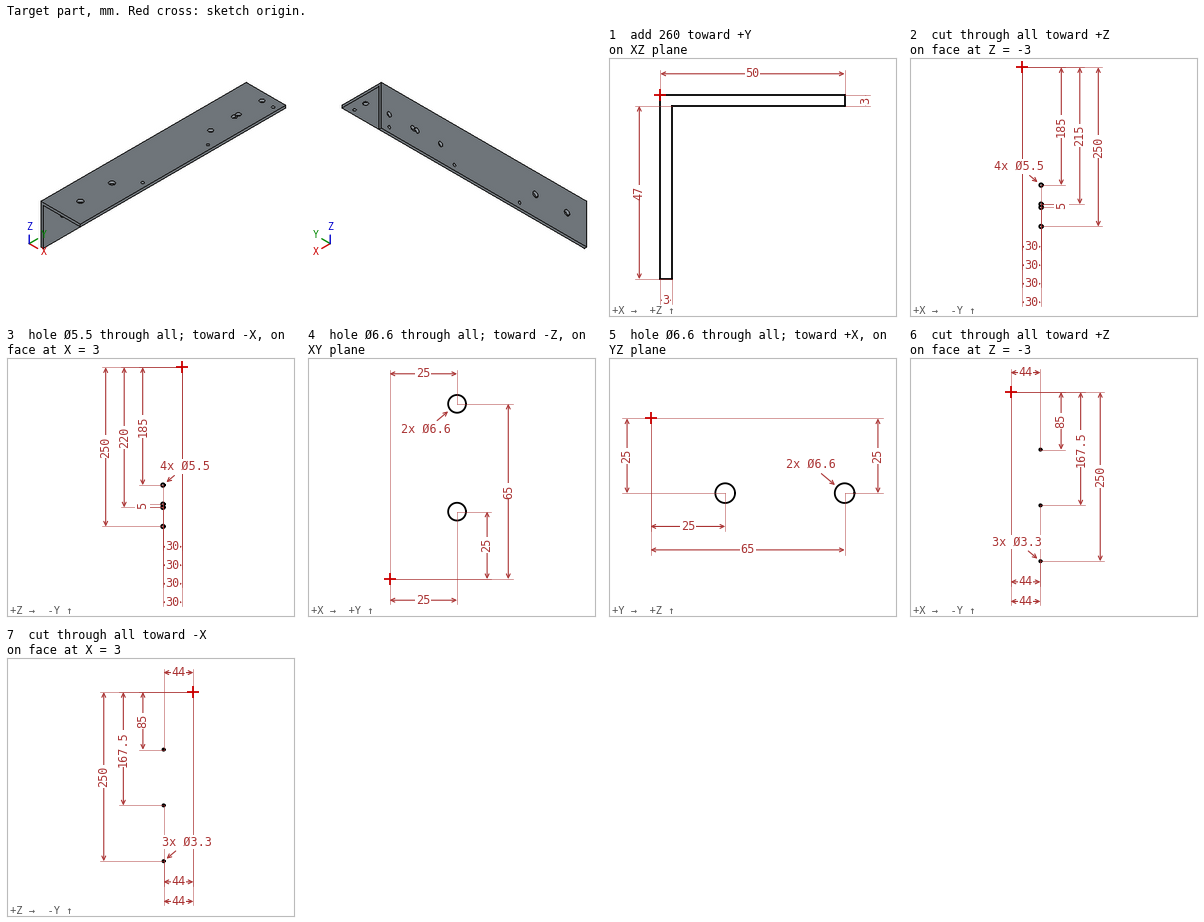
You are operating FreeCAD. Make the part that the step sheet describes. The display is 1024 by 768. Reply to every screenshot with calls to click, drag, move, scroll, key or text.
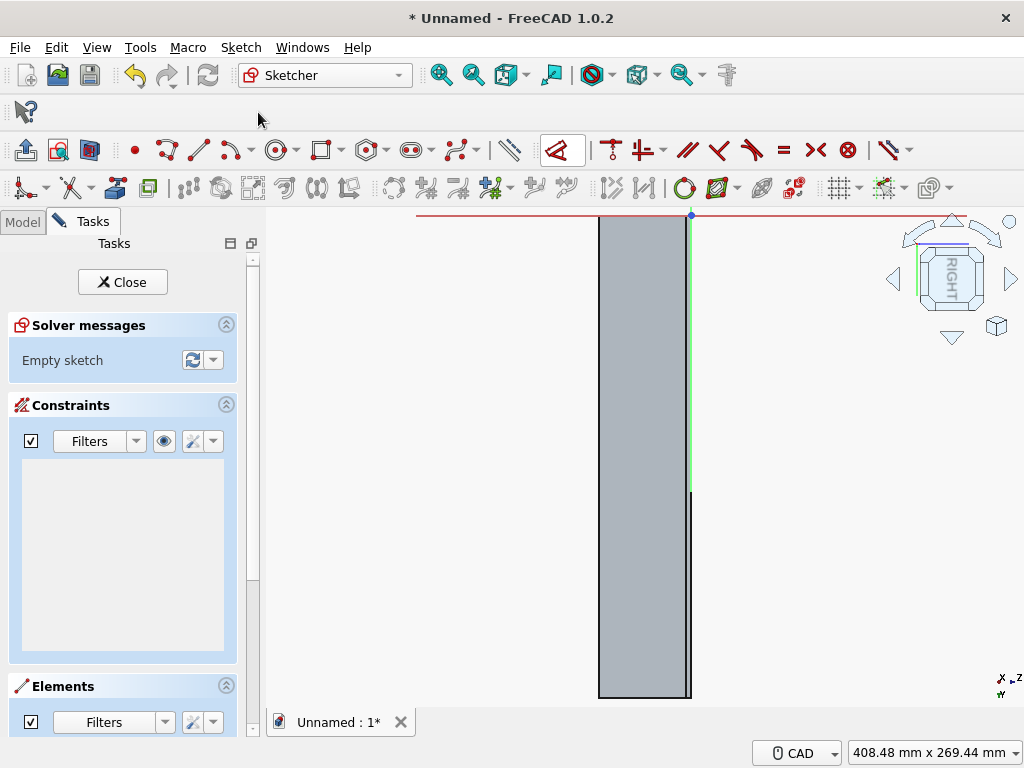
scroll(576, 457, down, 5)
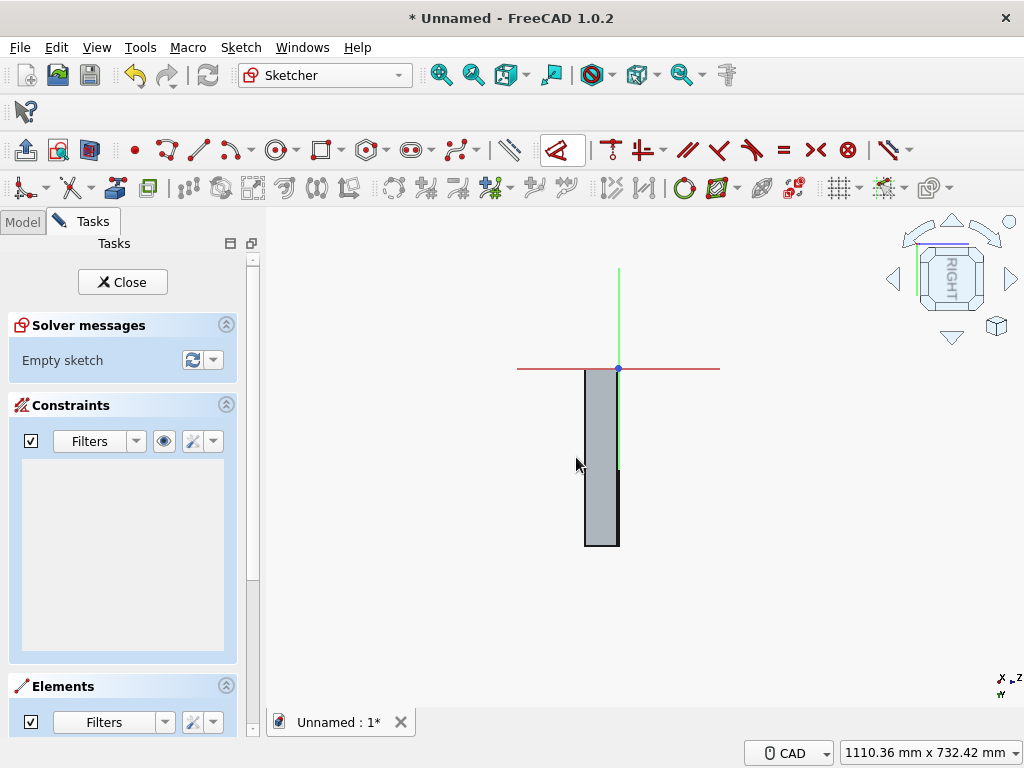
scroll(603, 529, up, 9)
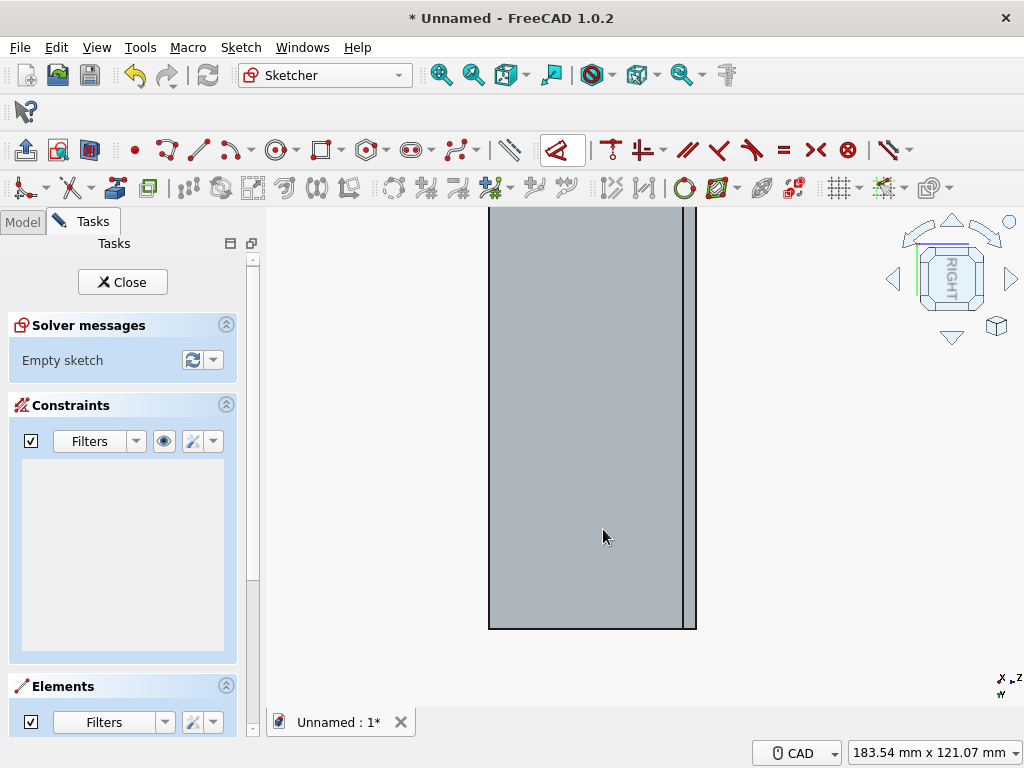
key(g)
key(c)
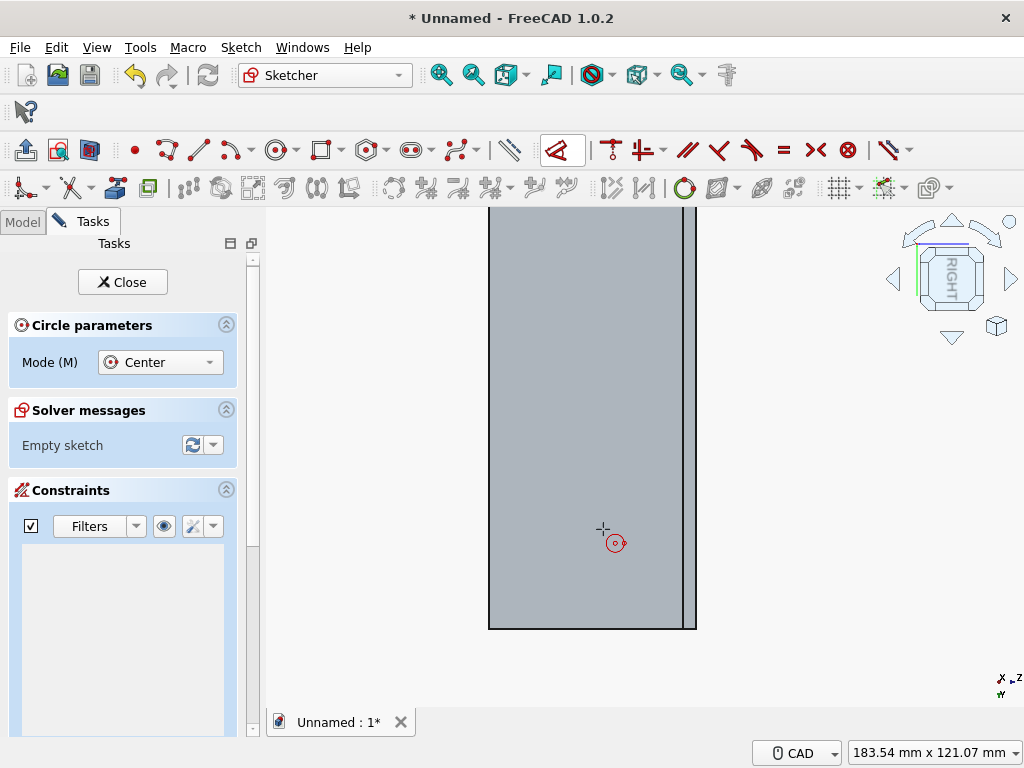
scroll(572, 464, up, 4)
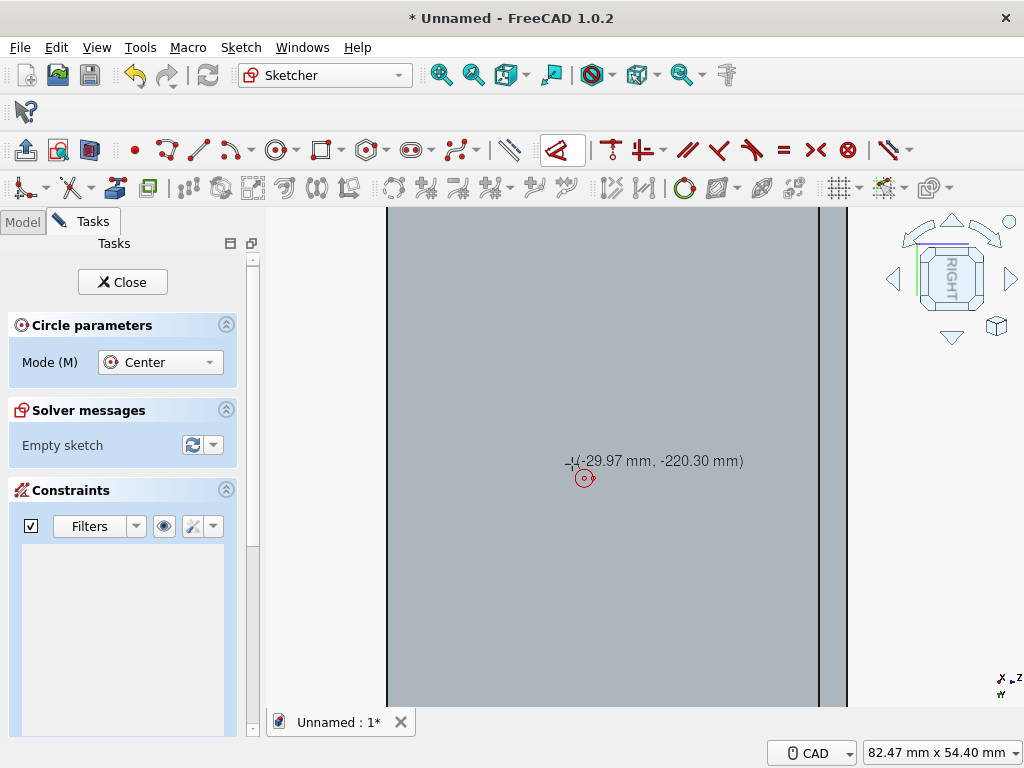
click(571, 463)
click(589, 445)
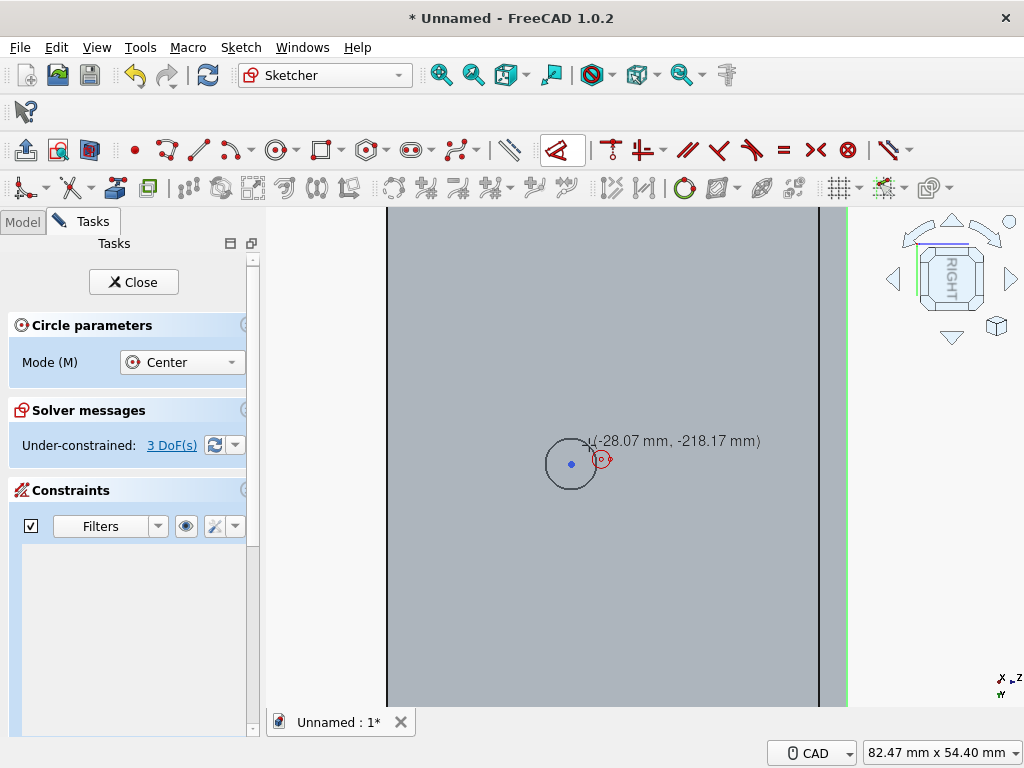
scroll(581, 471, down, 4)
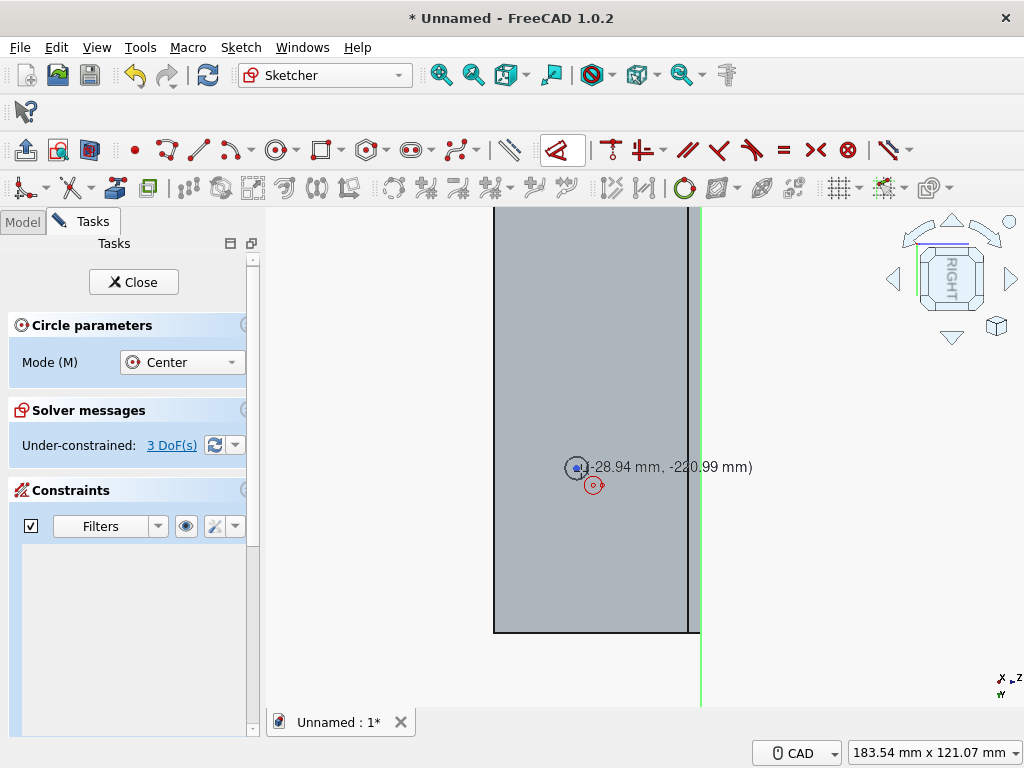
scroll(577, 323, up, 4)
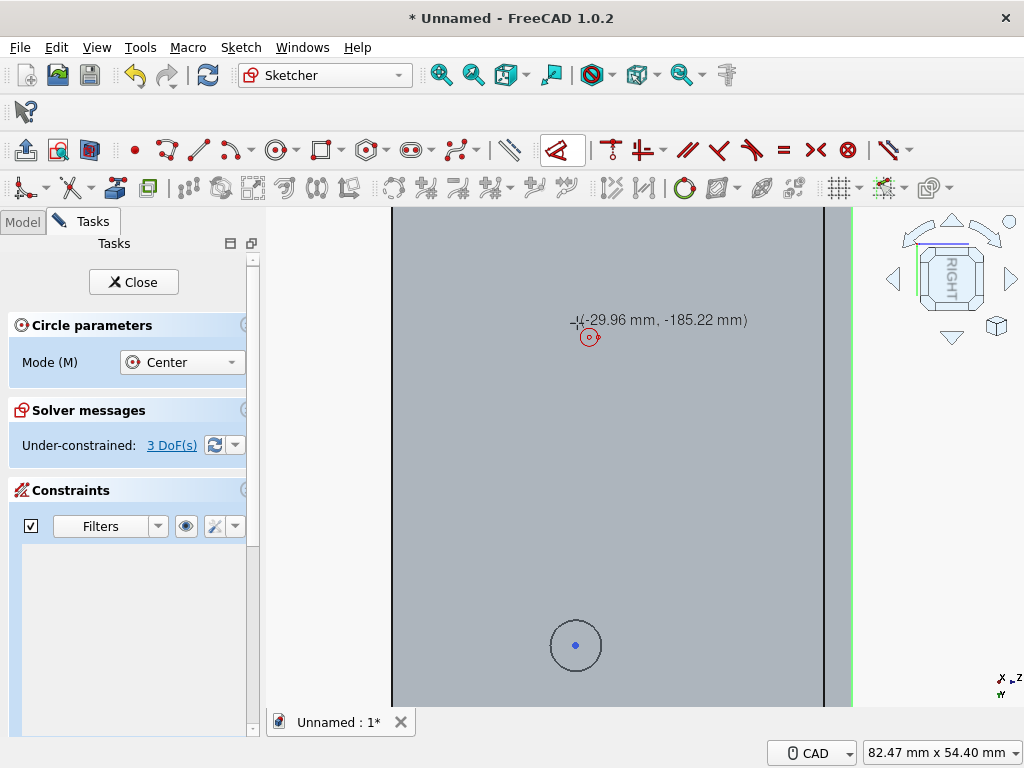
click(576, 323)
click(594, 305)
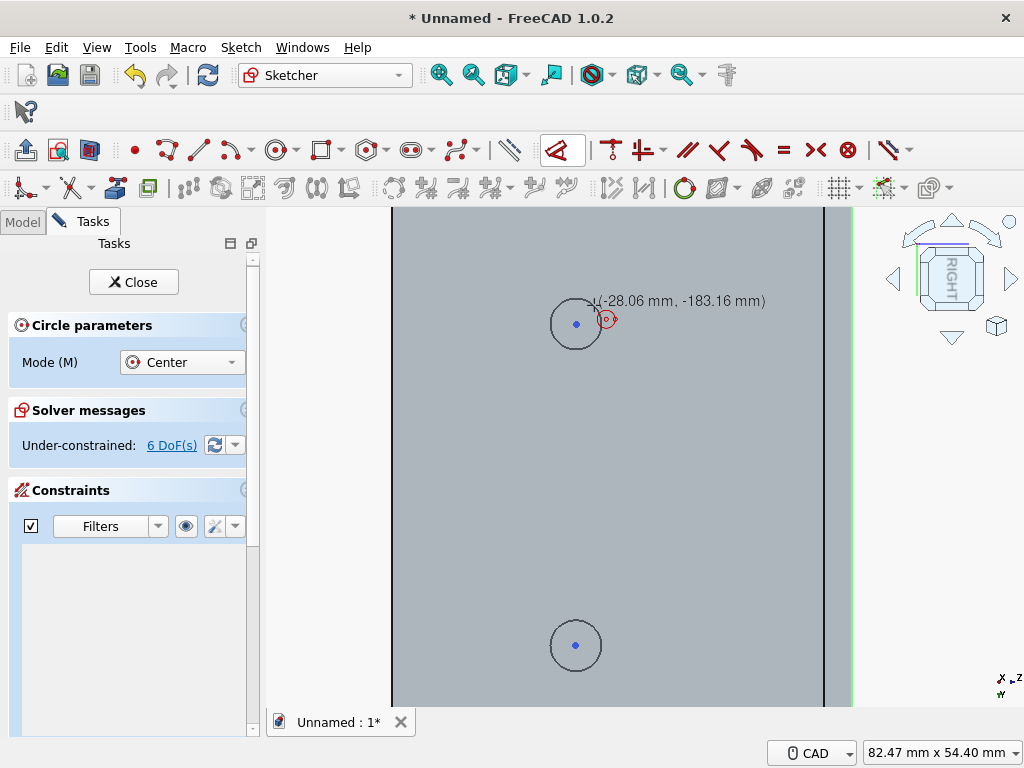
scroll(577, 323, down, 4)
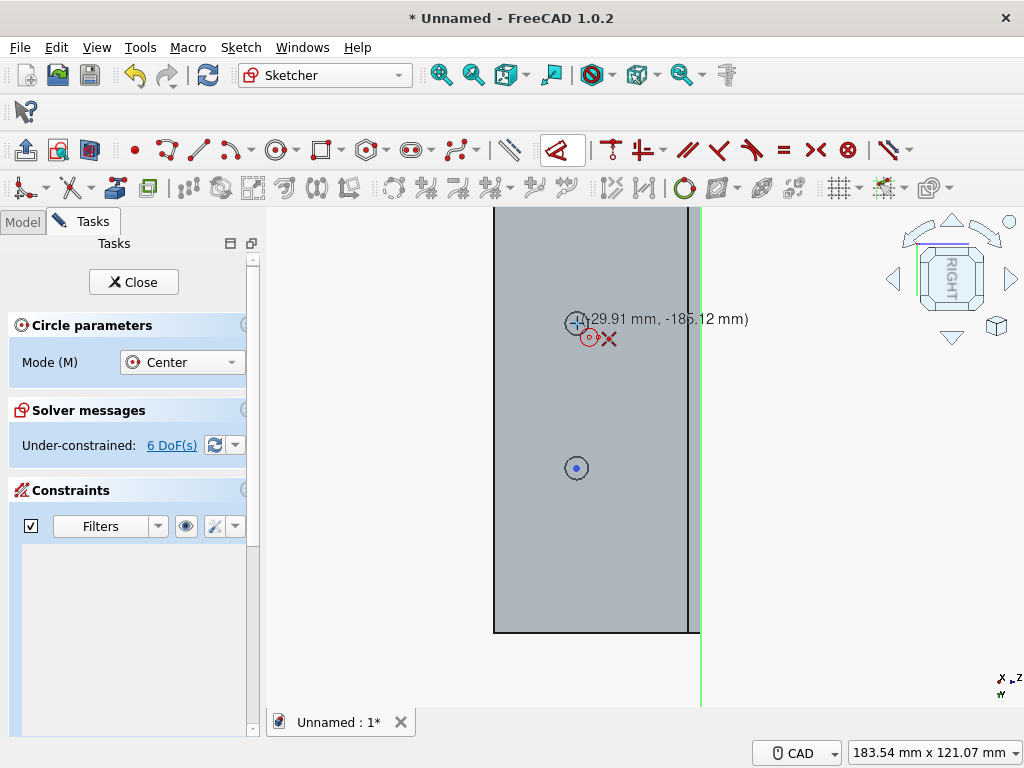
scroll(577, 592, up, 4)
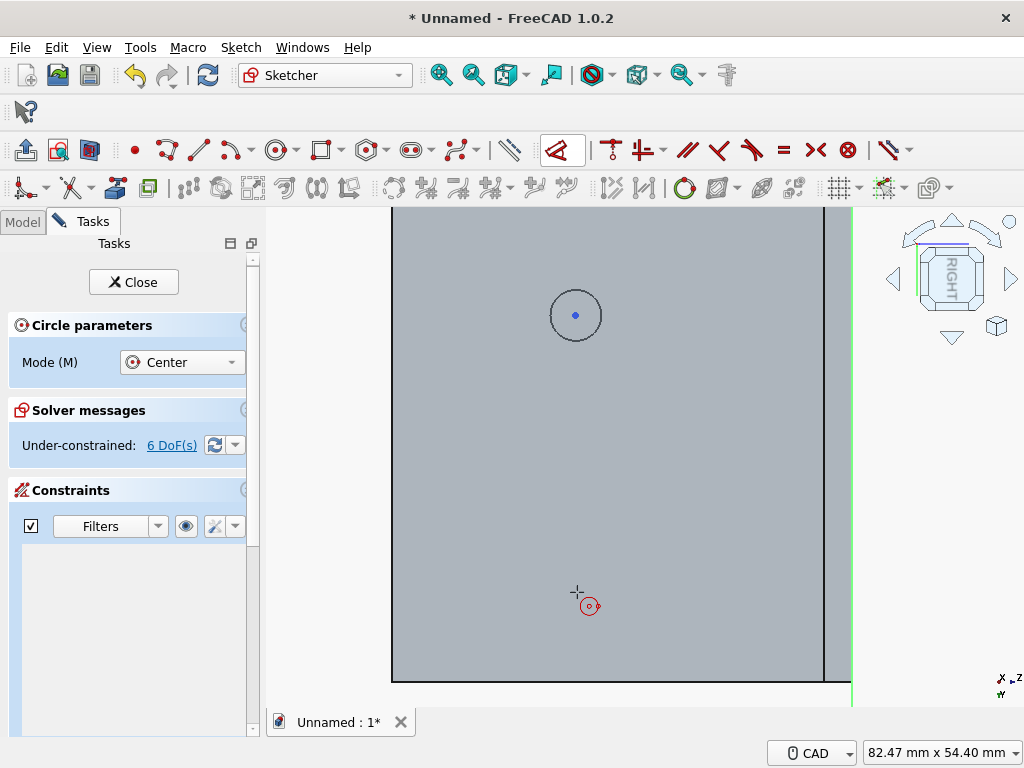
click(576, 590)
click(594, 572)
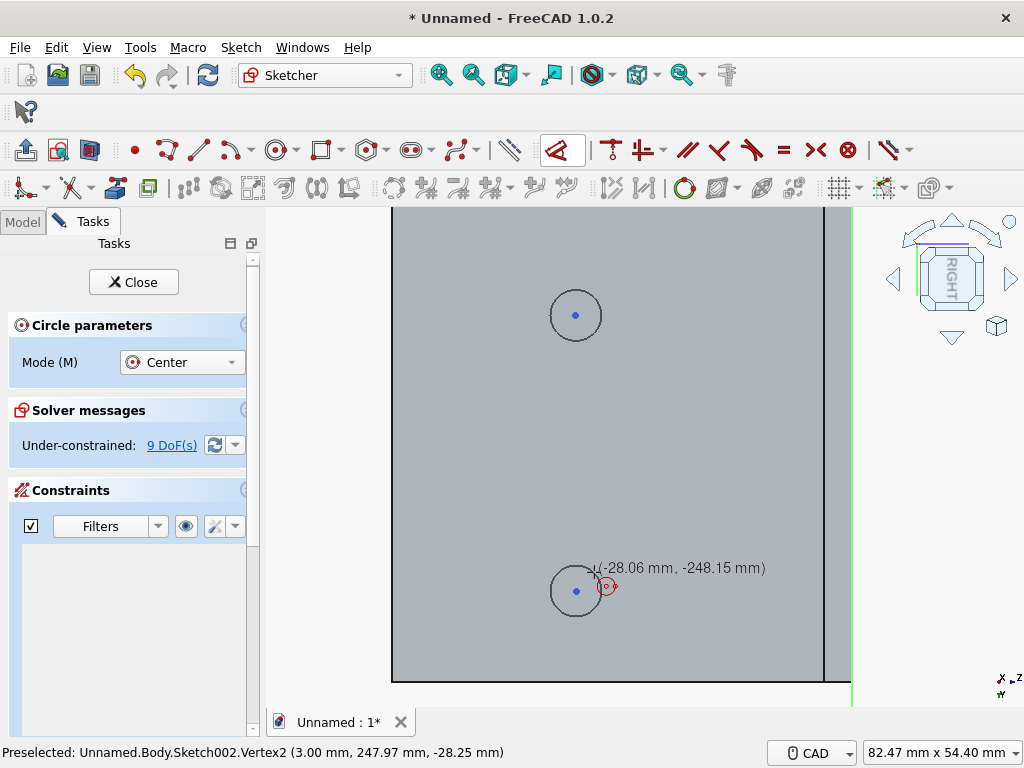
click(576, 268)
click(594, 250)
key(Escape)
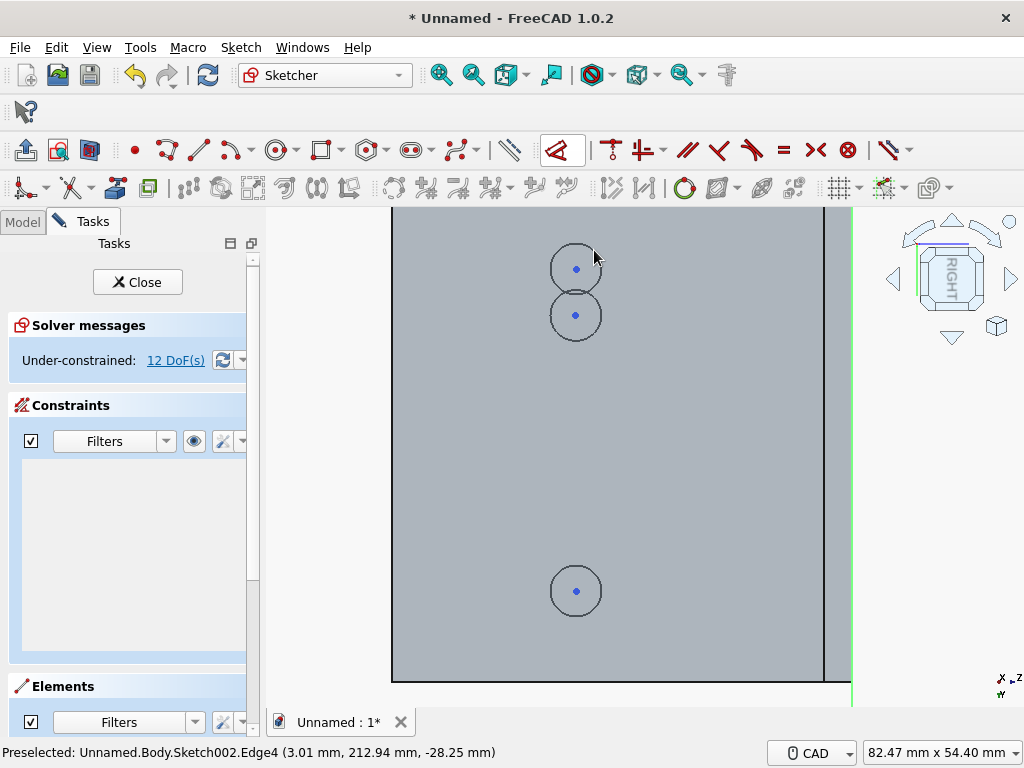
click(558, 333)